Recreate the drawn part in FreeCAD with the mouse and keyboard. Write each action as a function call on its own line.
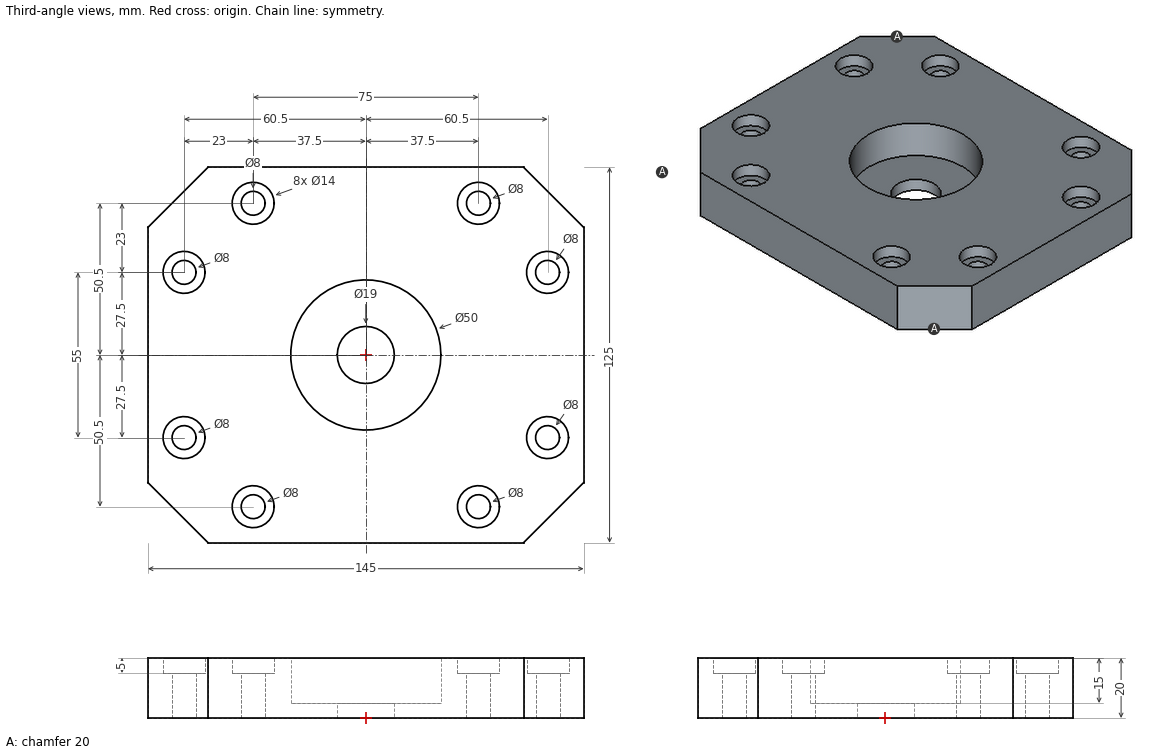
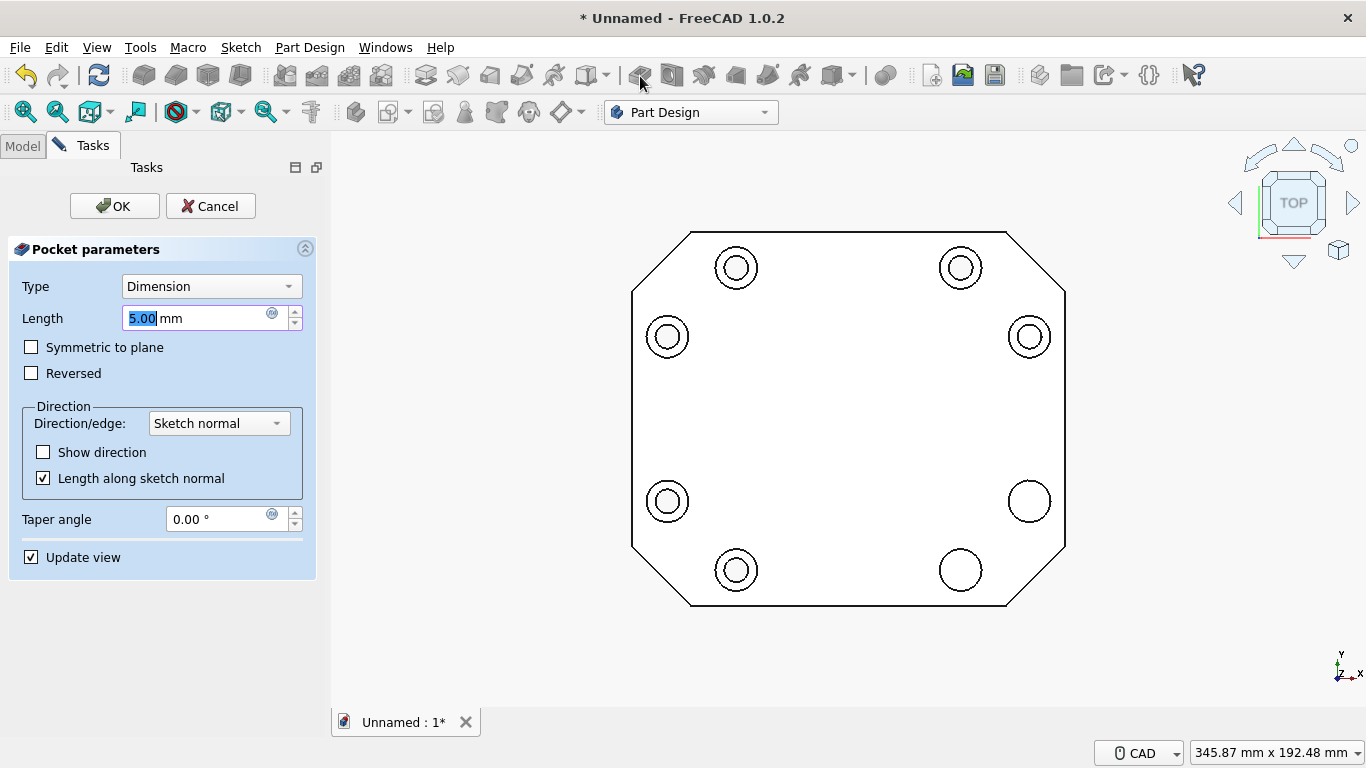
click(212, 286)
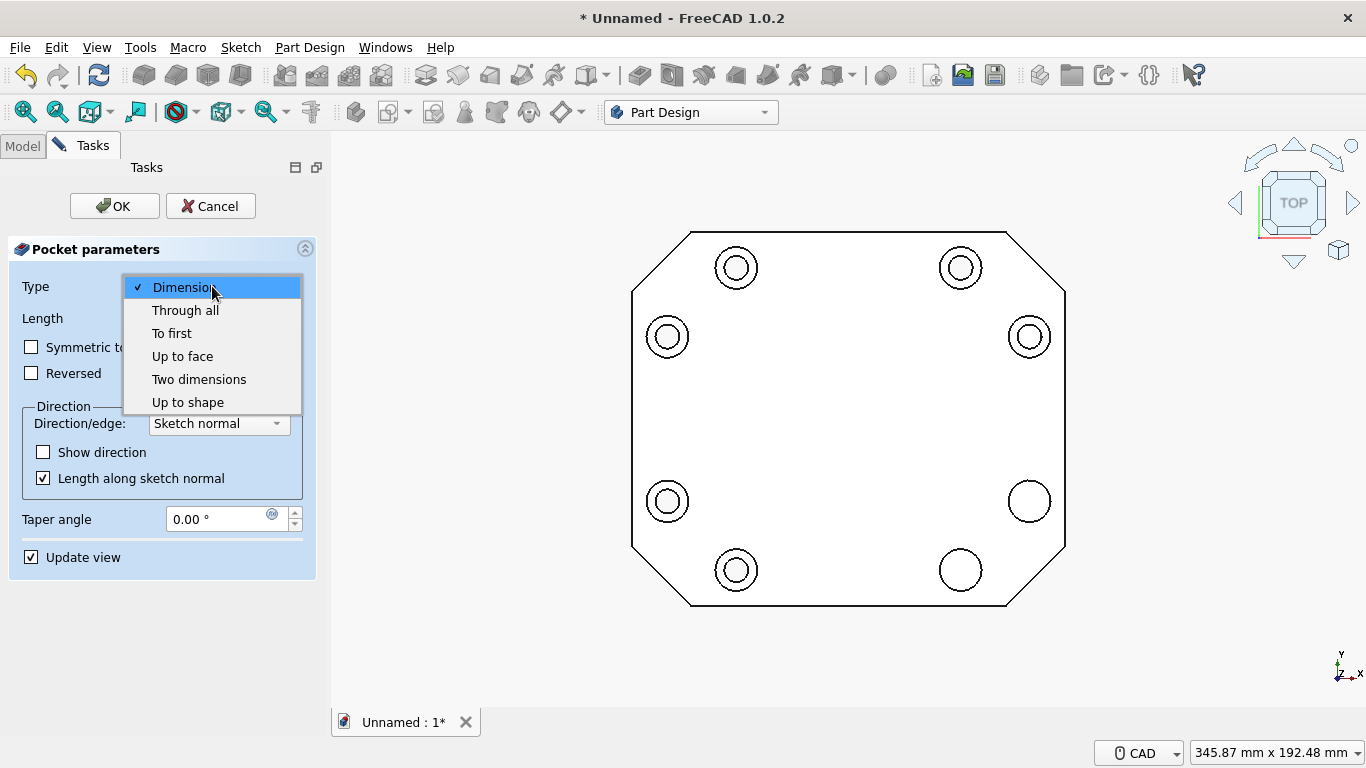
click(212, 334)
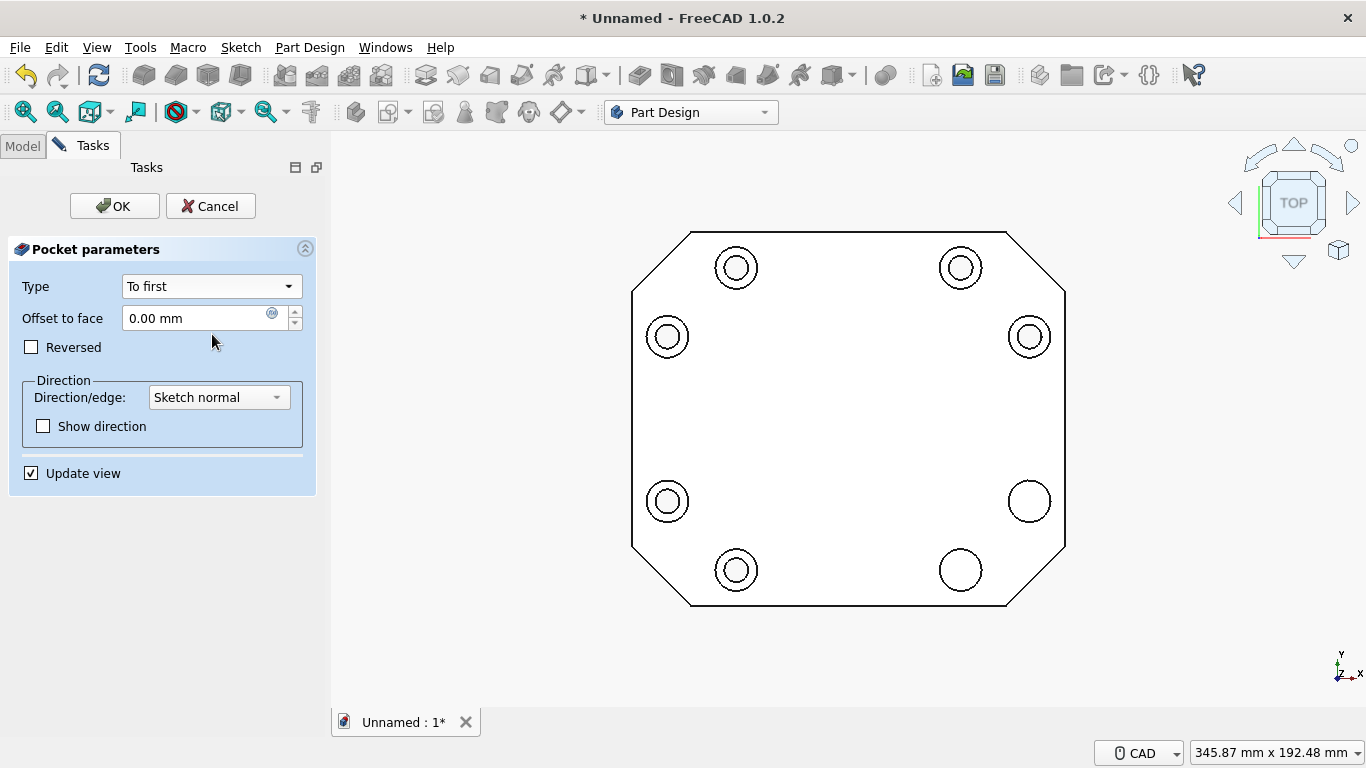
click(115, 206)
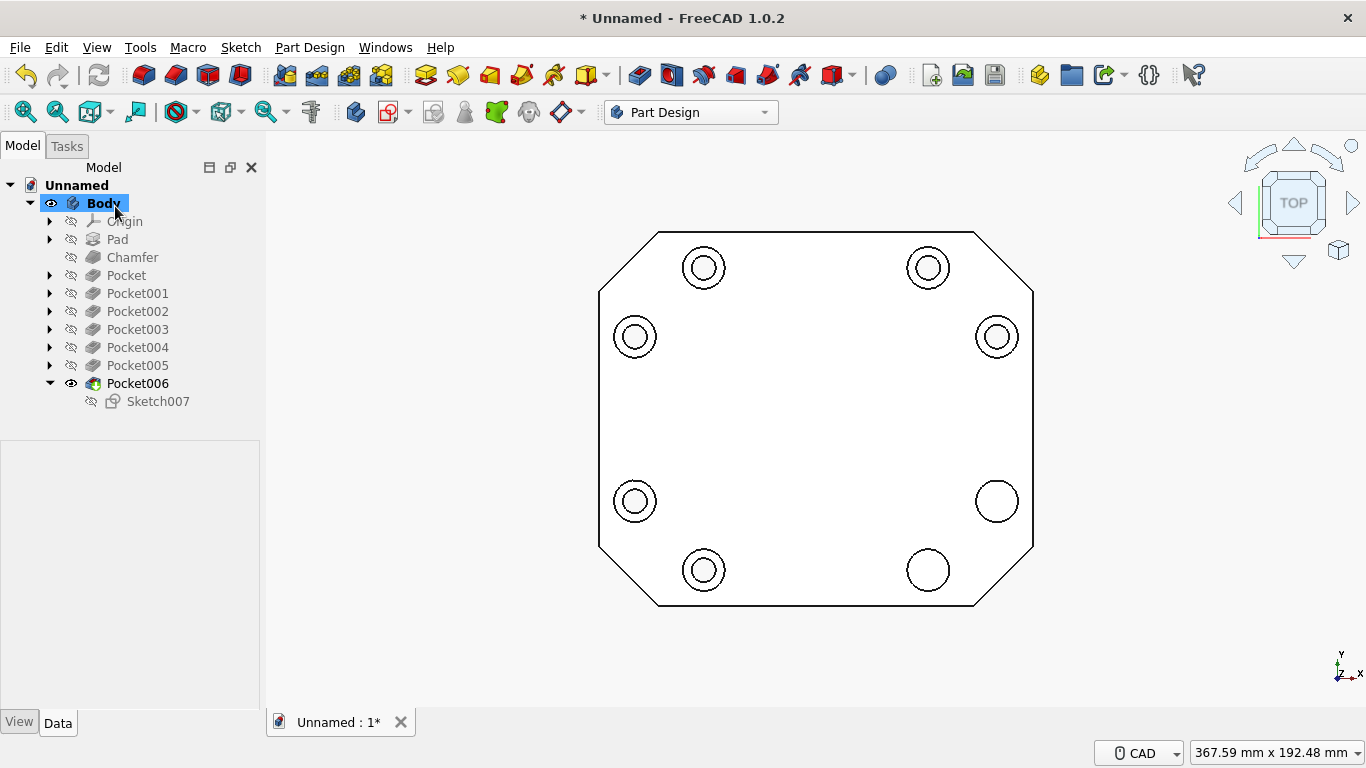
click(928, 569)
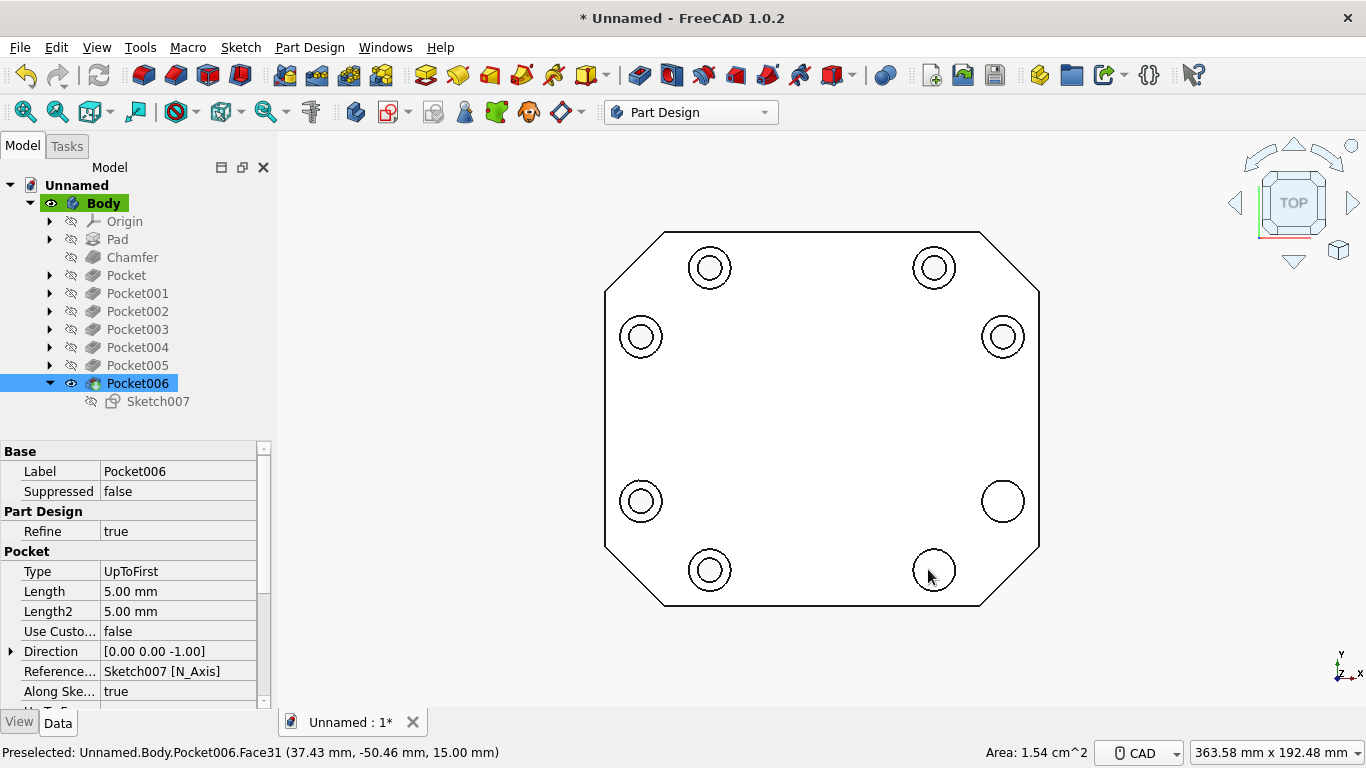
click(388, 112)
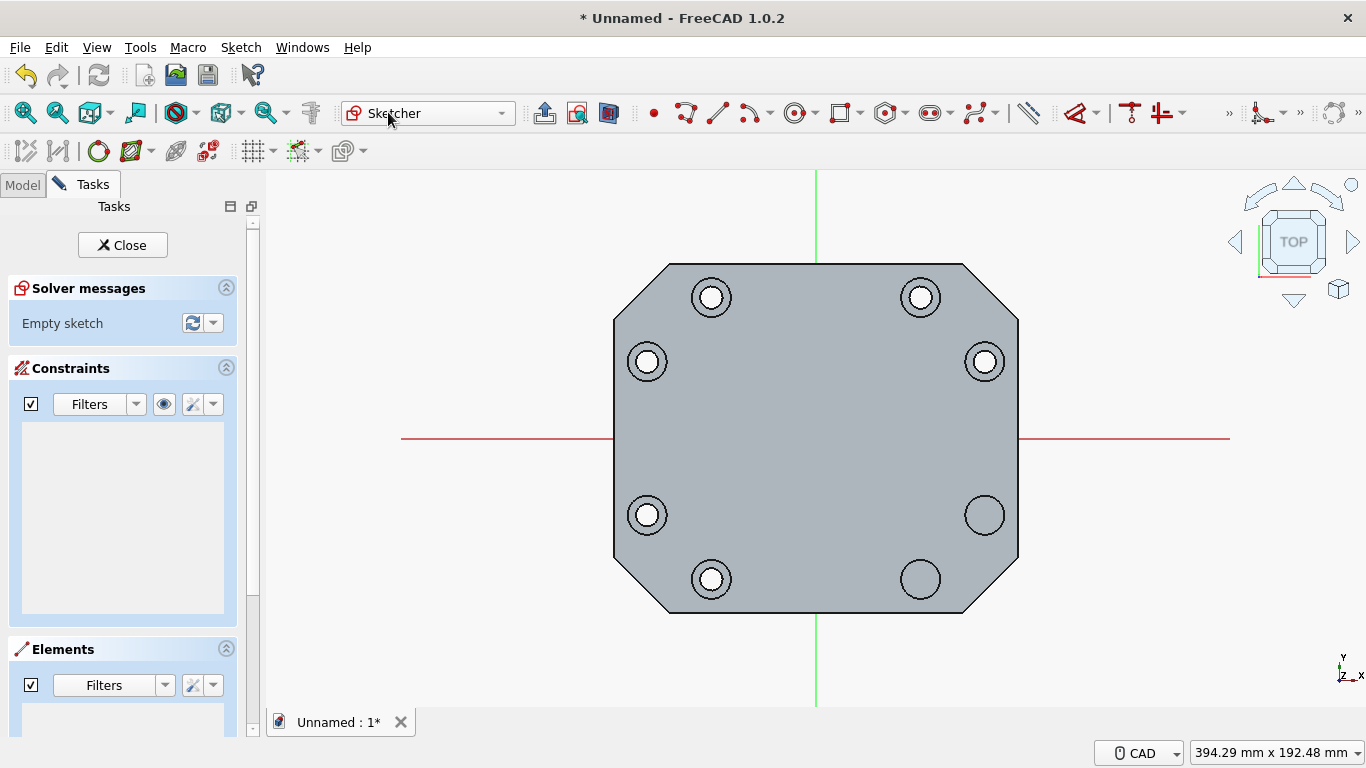
scroll(1000, 520, up, 14)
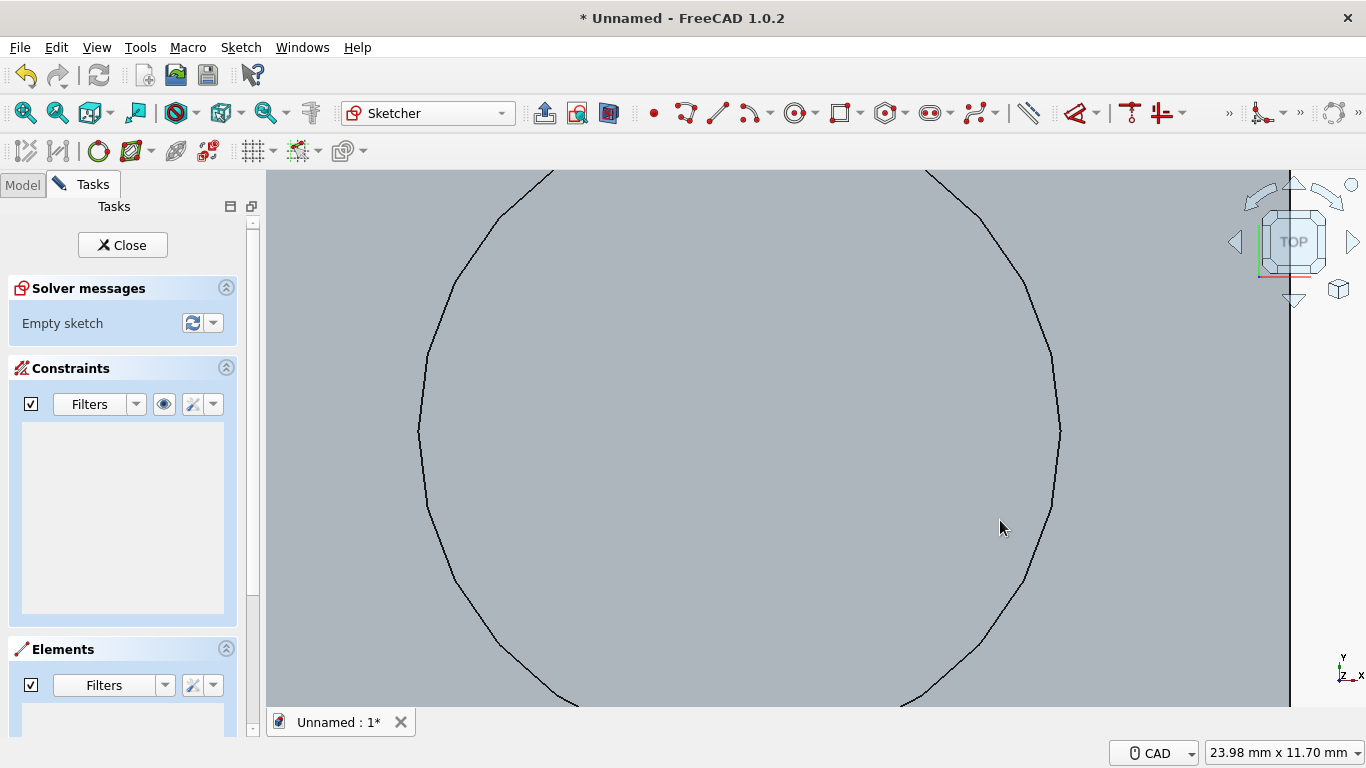
click(796, 114)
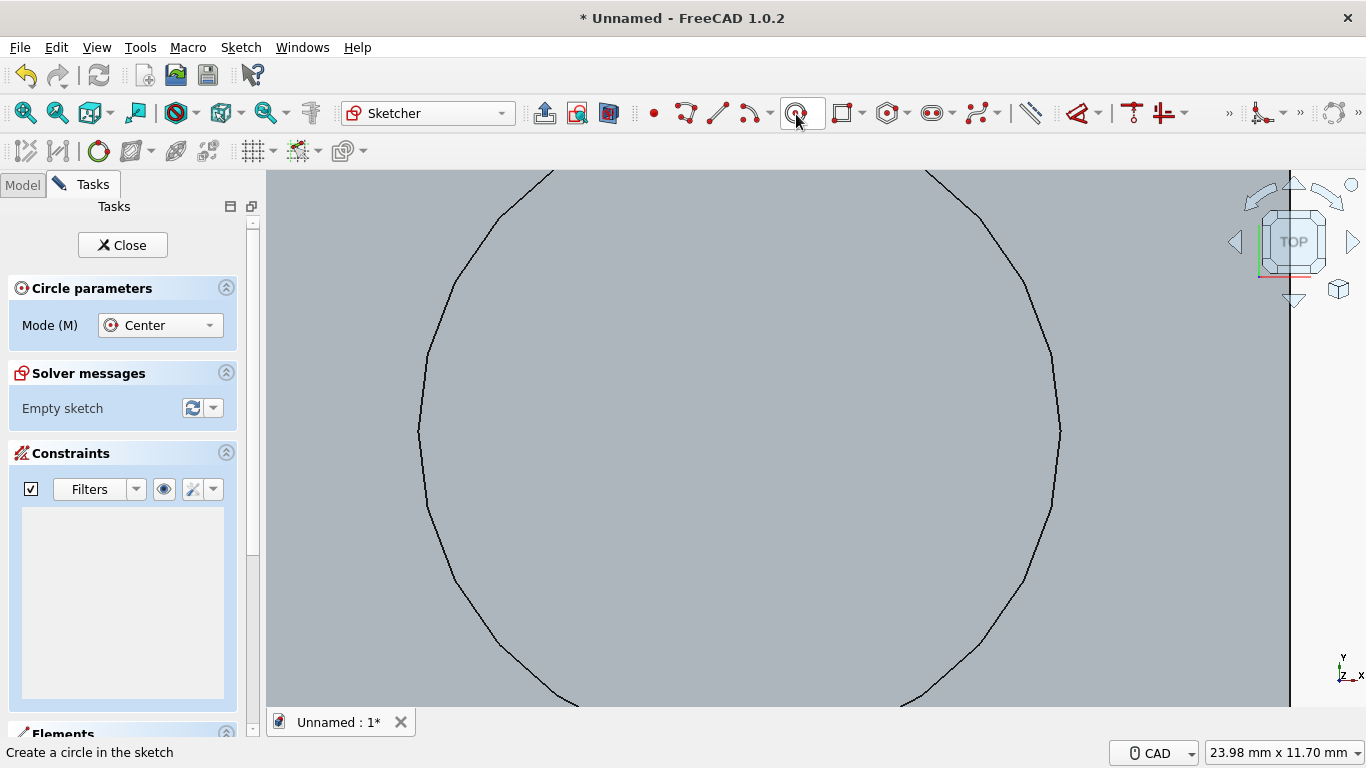
click(739, 431)
click(869, 302)
key(Escape)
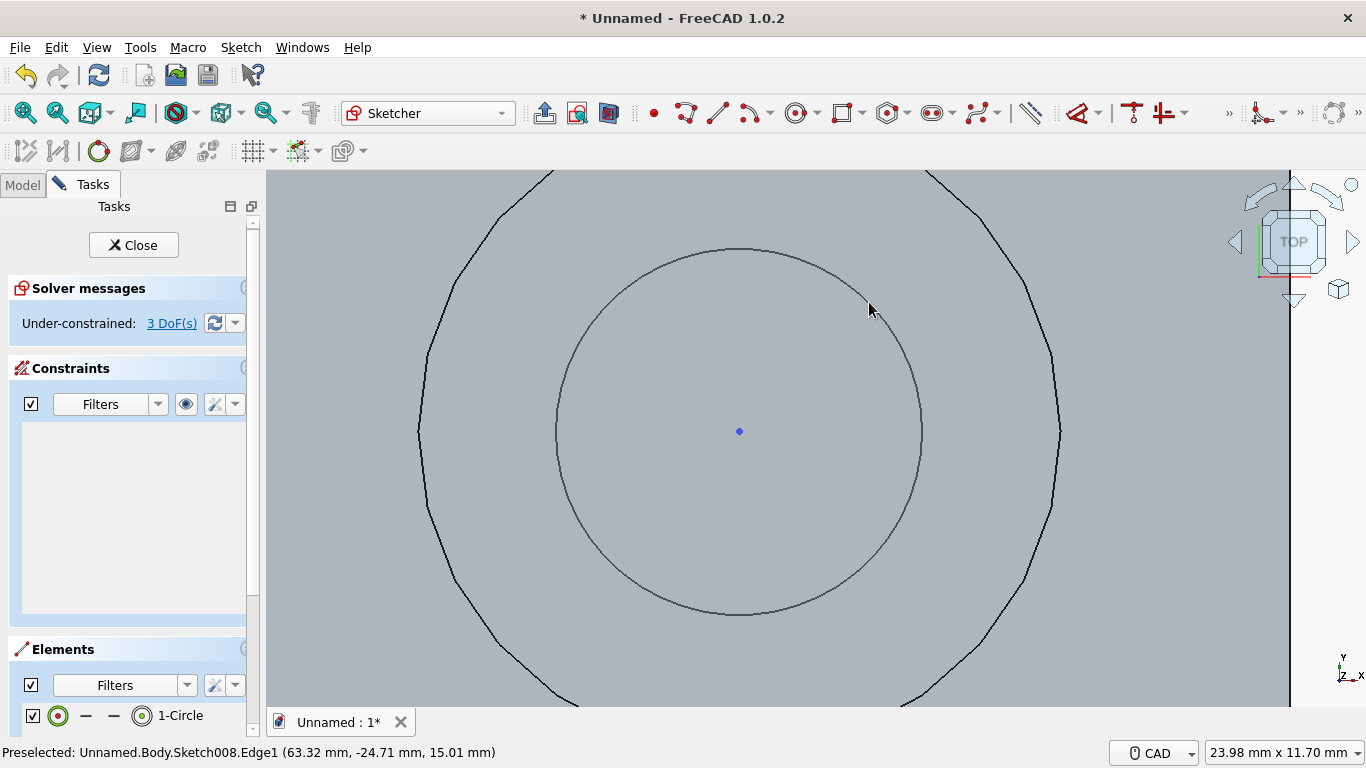
click(1078, 114)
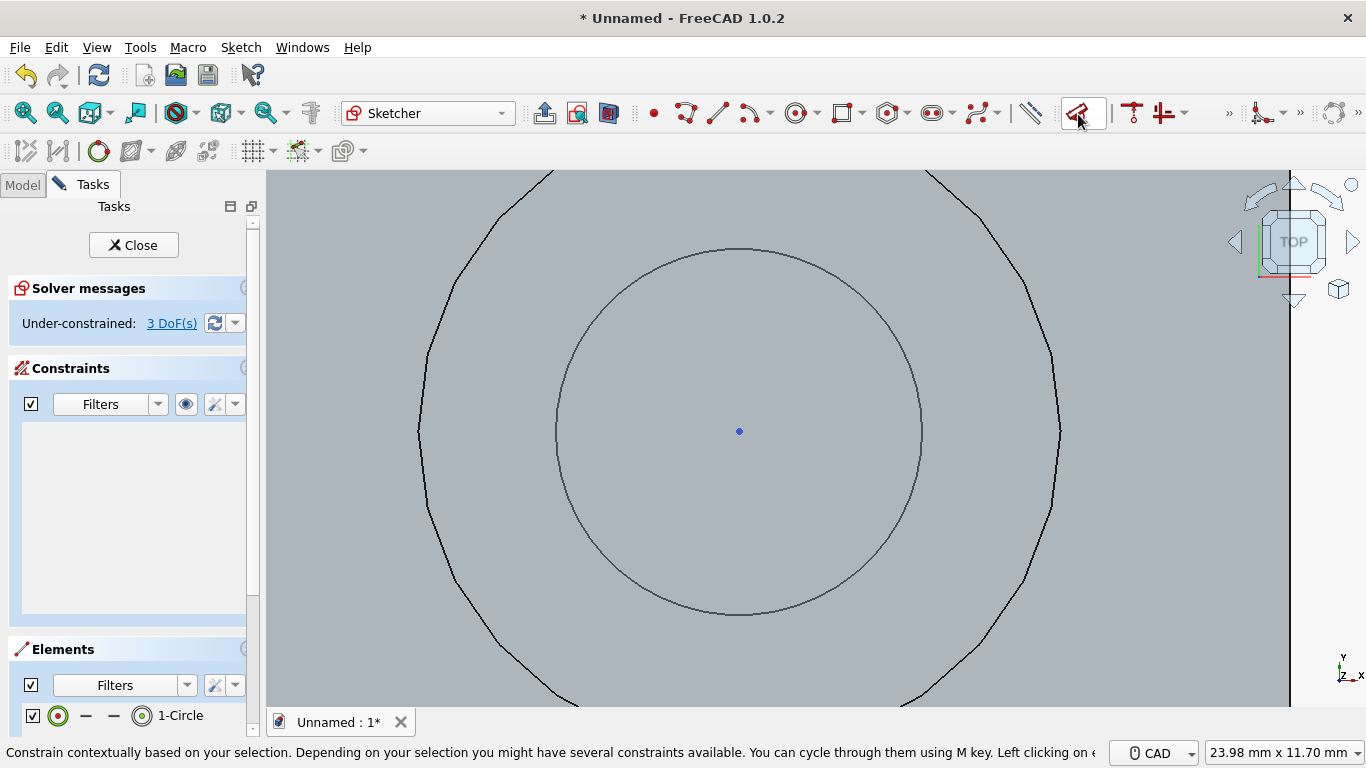
click(868, 302)
click(891, 279)